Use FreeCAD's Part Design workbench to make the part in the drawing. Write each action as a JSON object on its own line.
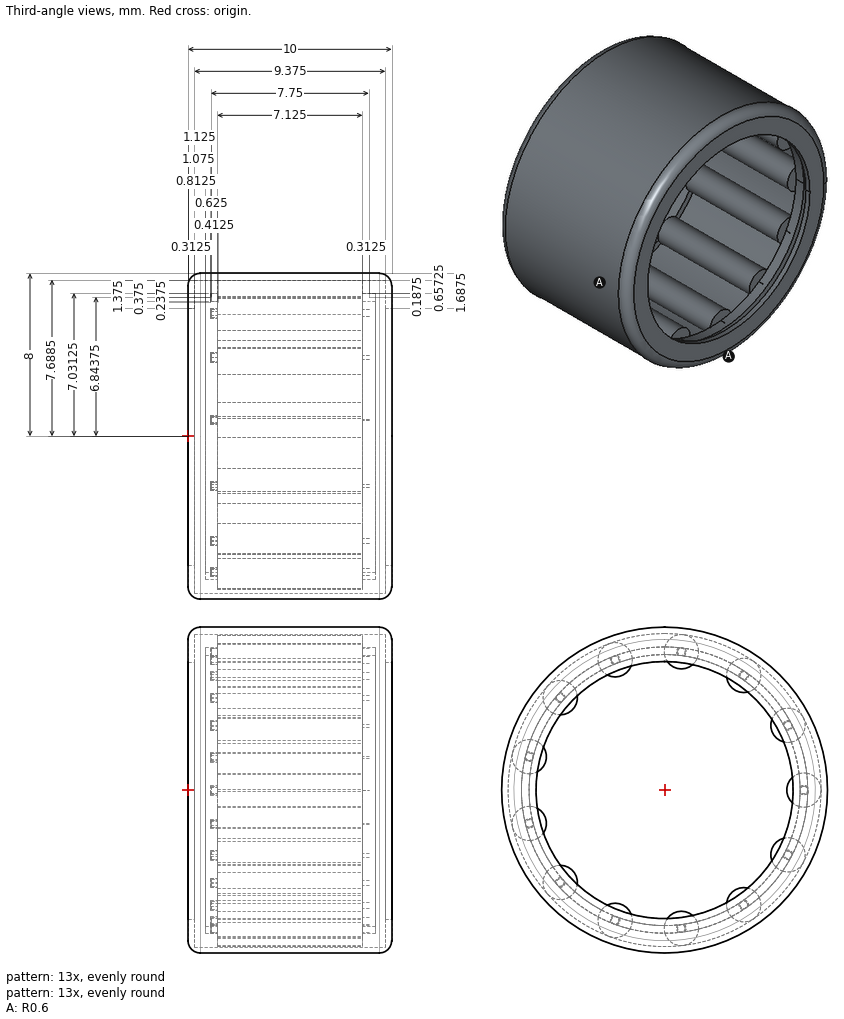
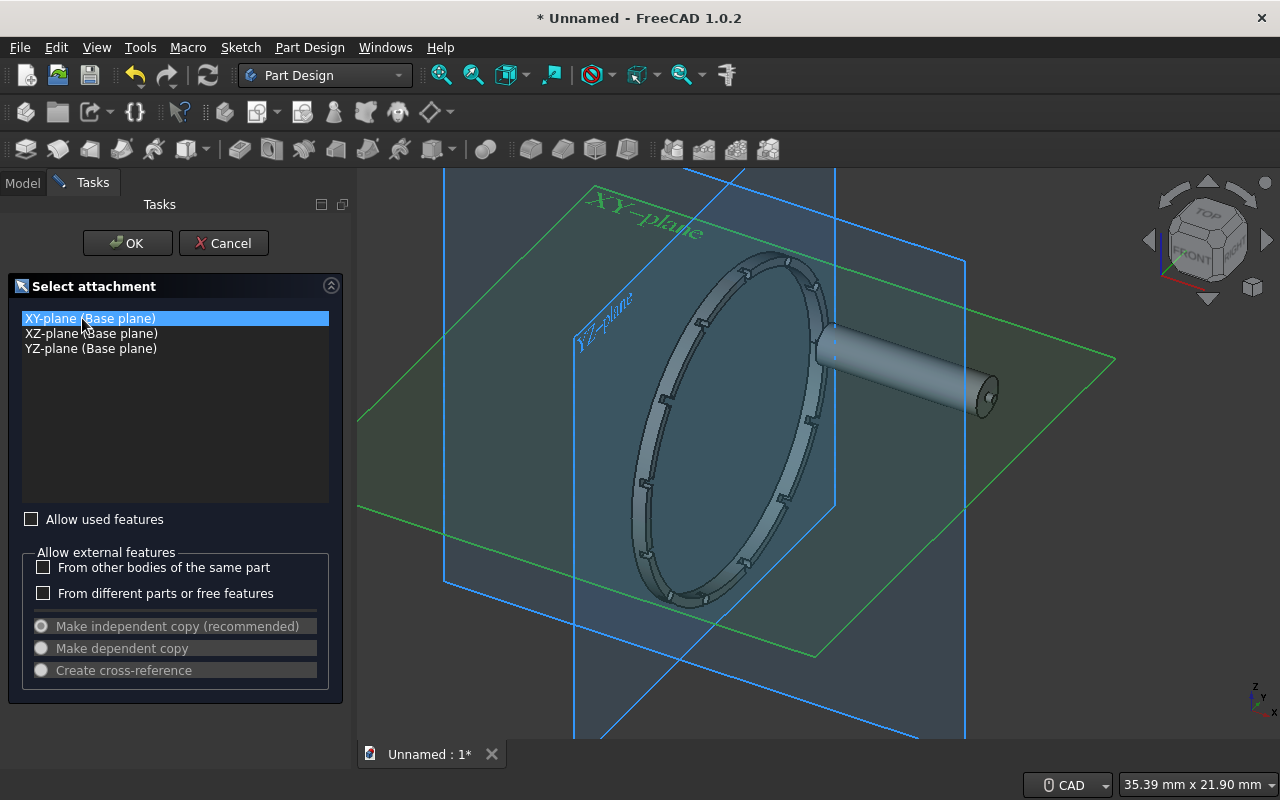
{"action": "left_click", "coordinate": [128, 243]}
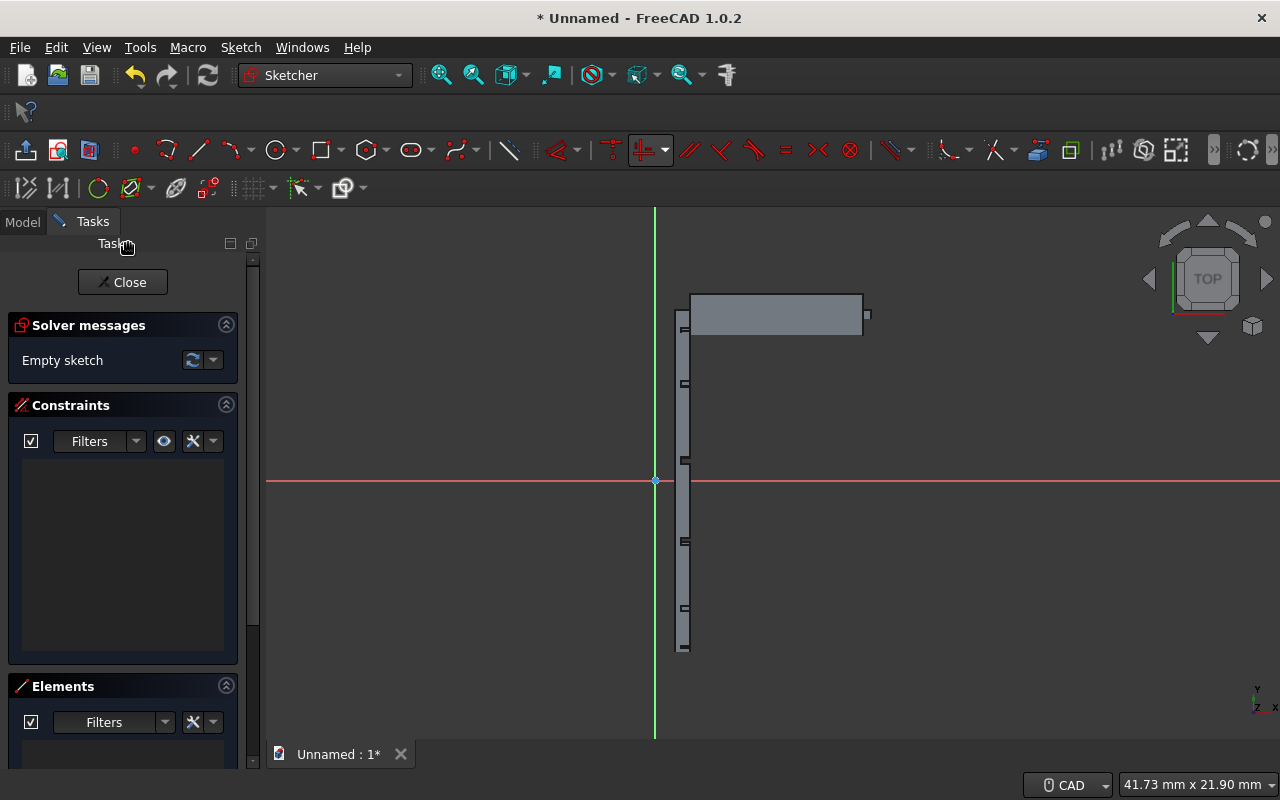
{"action": "left_click", "coordinate": [90, 150]}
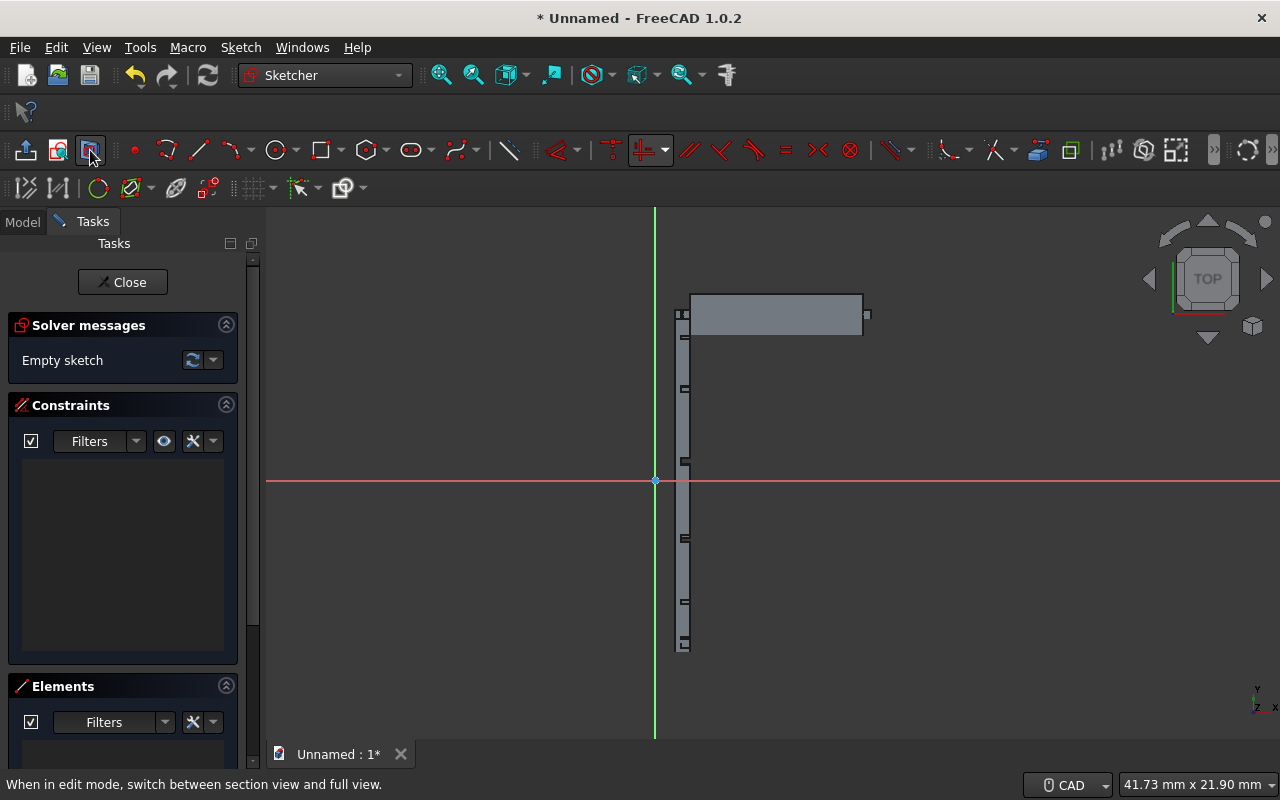
{"action": "scroll", "coordinate": [865, 275], "scroll_direction": "up", "scroll_amount": 3}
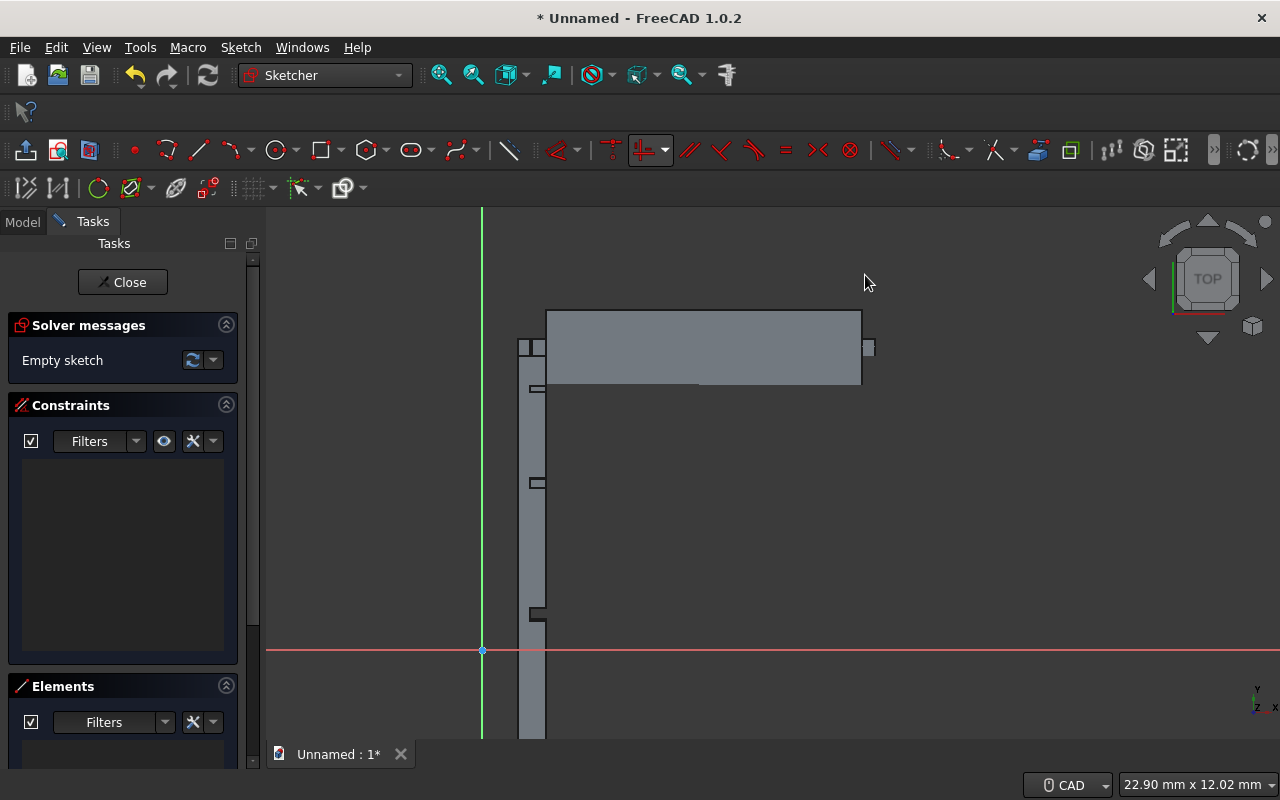
{"action": "left_click", "coordinate": [168, 150]}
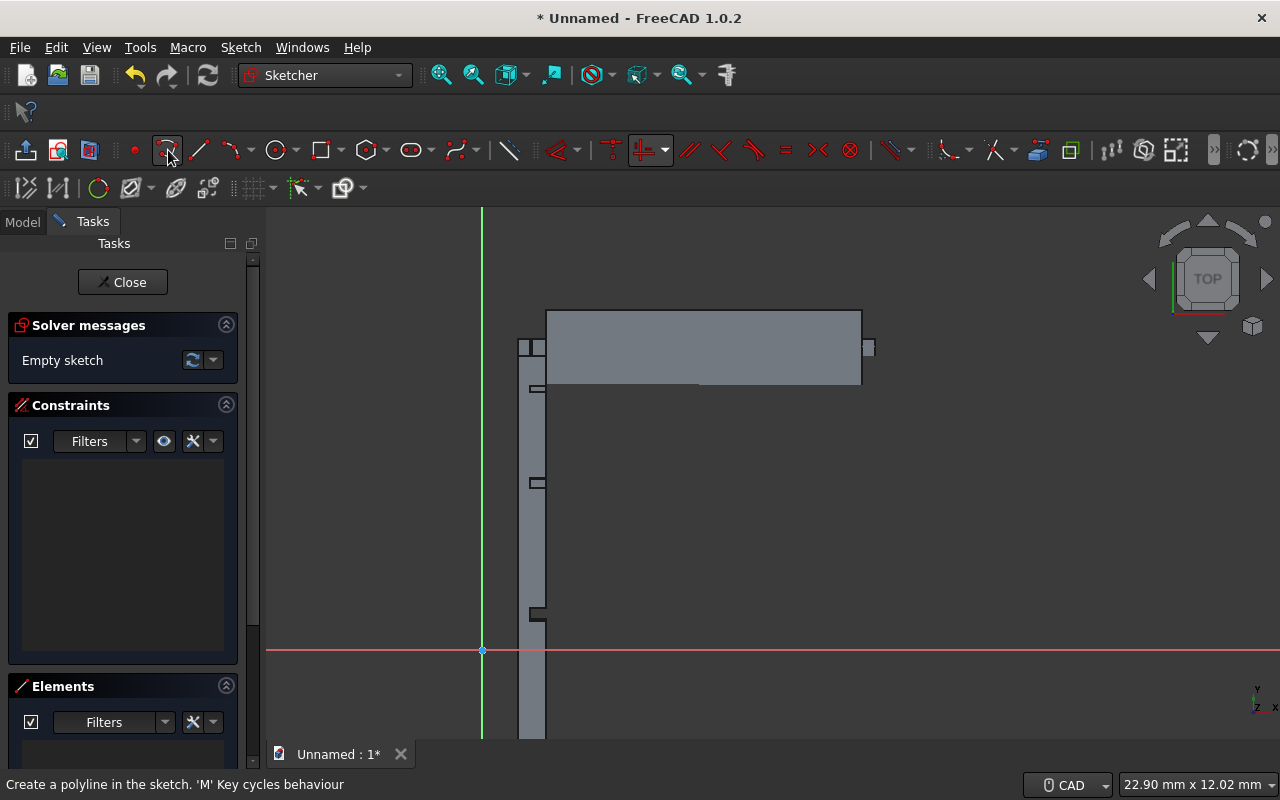
{"action": "left_click", "coordinate": [482, 371]}
{"action": "left_click", "coordinate": [496, 371]}
{"action": "left_click", "coordinate": [496, 310]}
{"action": "left_click", "coordinate": [911, 310]}
{"action": "left_click", "coordinate": [911, 371]}
{"action": "left_click", "coordinate": [925, 371]}
{"action": "left_click", "coordinate": [925, 296]}
{"action": "left_click", "coordinate": [491, 296]}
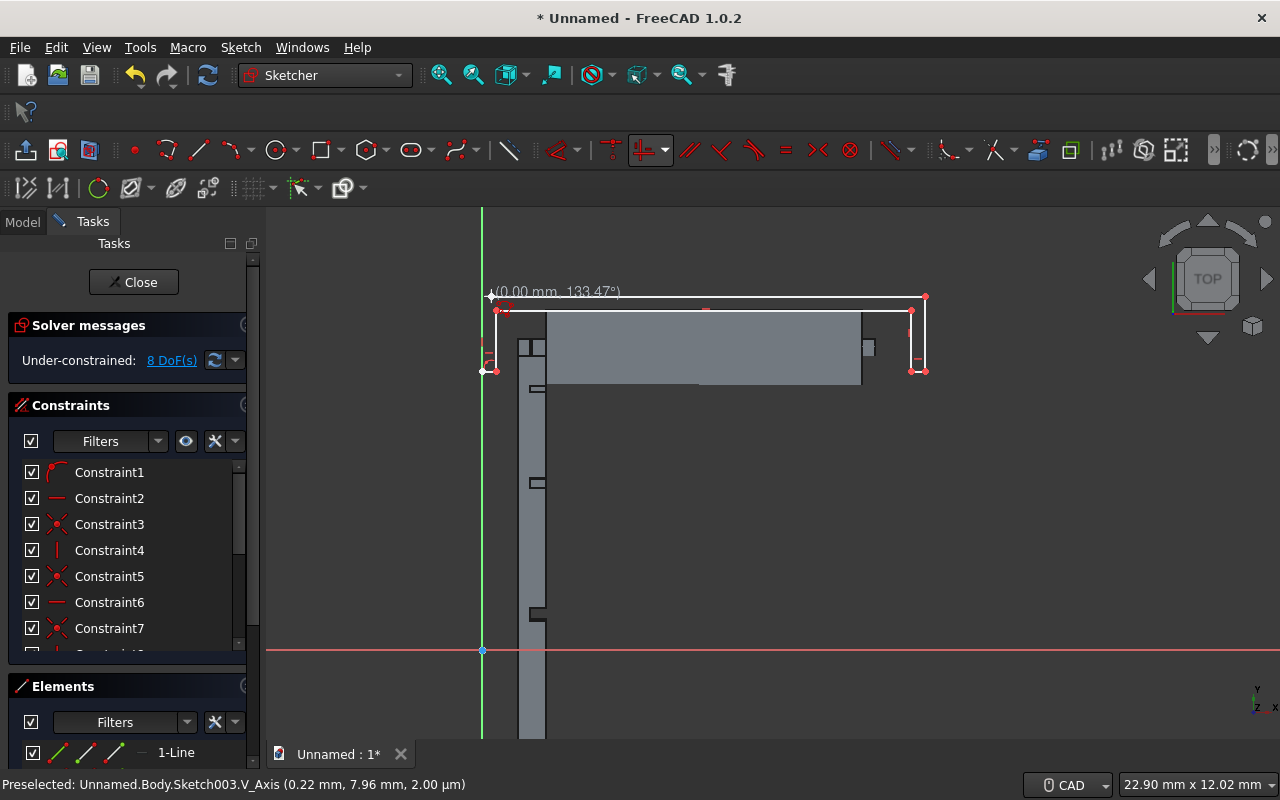
{"action": "scroll", "coordinate": [482, 371], "scroll_direction": "up", "scroll_amount": 5}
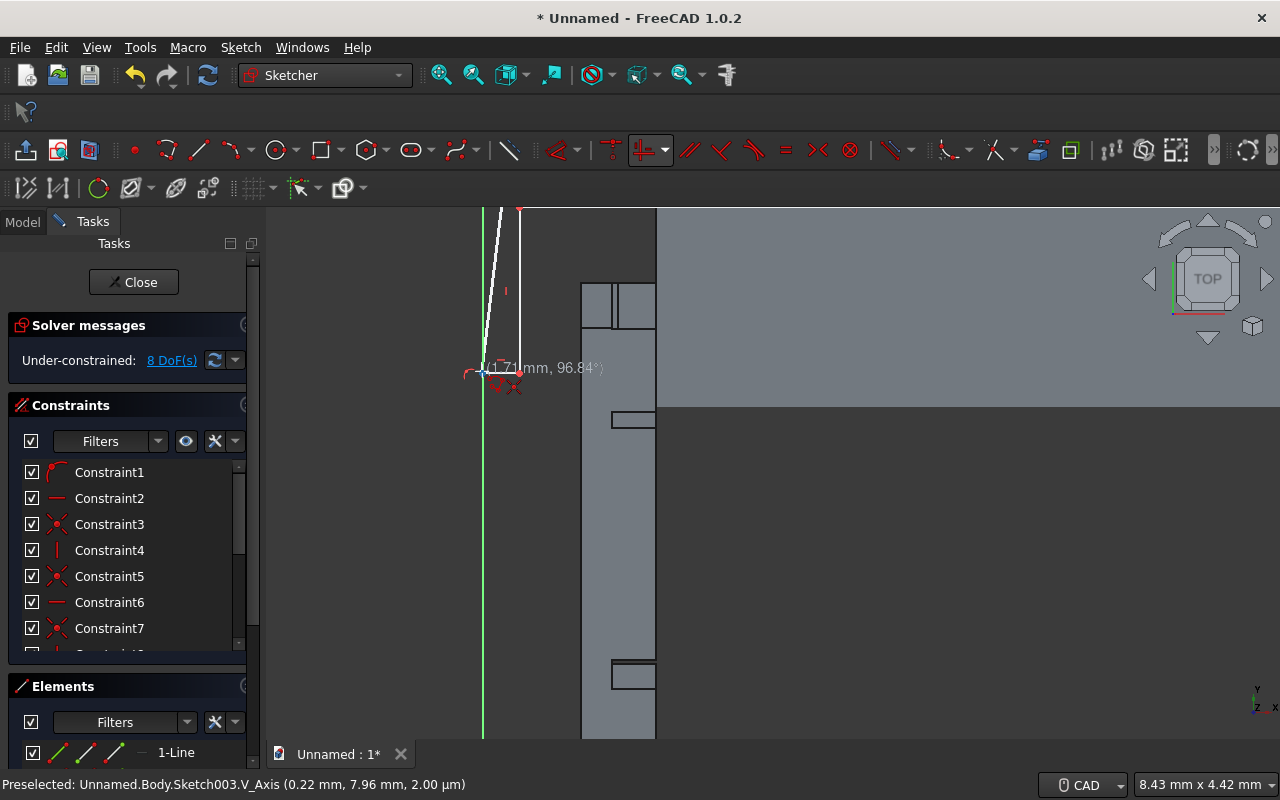
{"action": "left_click", "coordinate": [483, 373]}
{"action": "key", "text": "Escape"}
{"action": "key", "text": "Escape"}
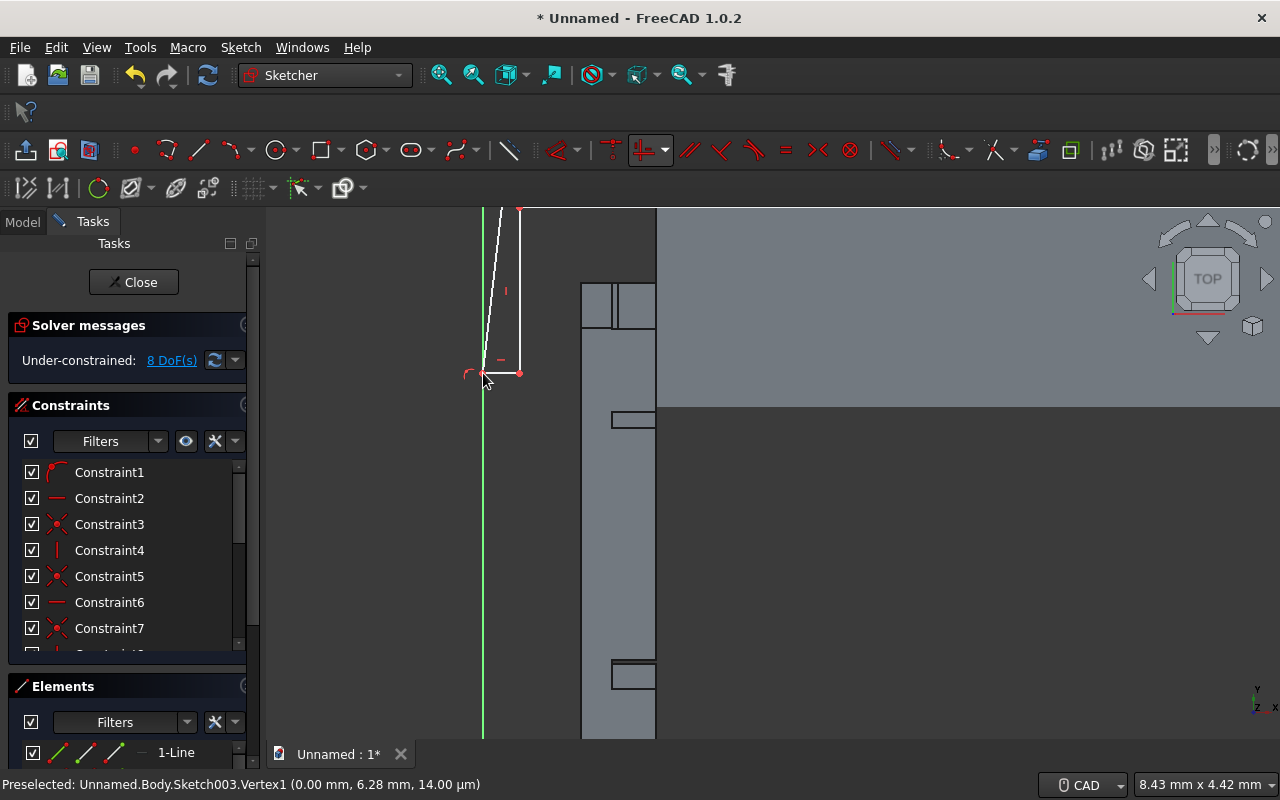
{"action": "left_click", "coordinate": [497, 251]}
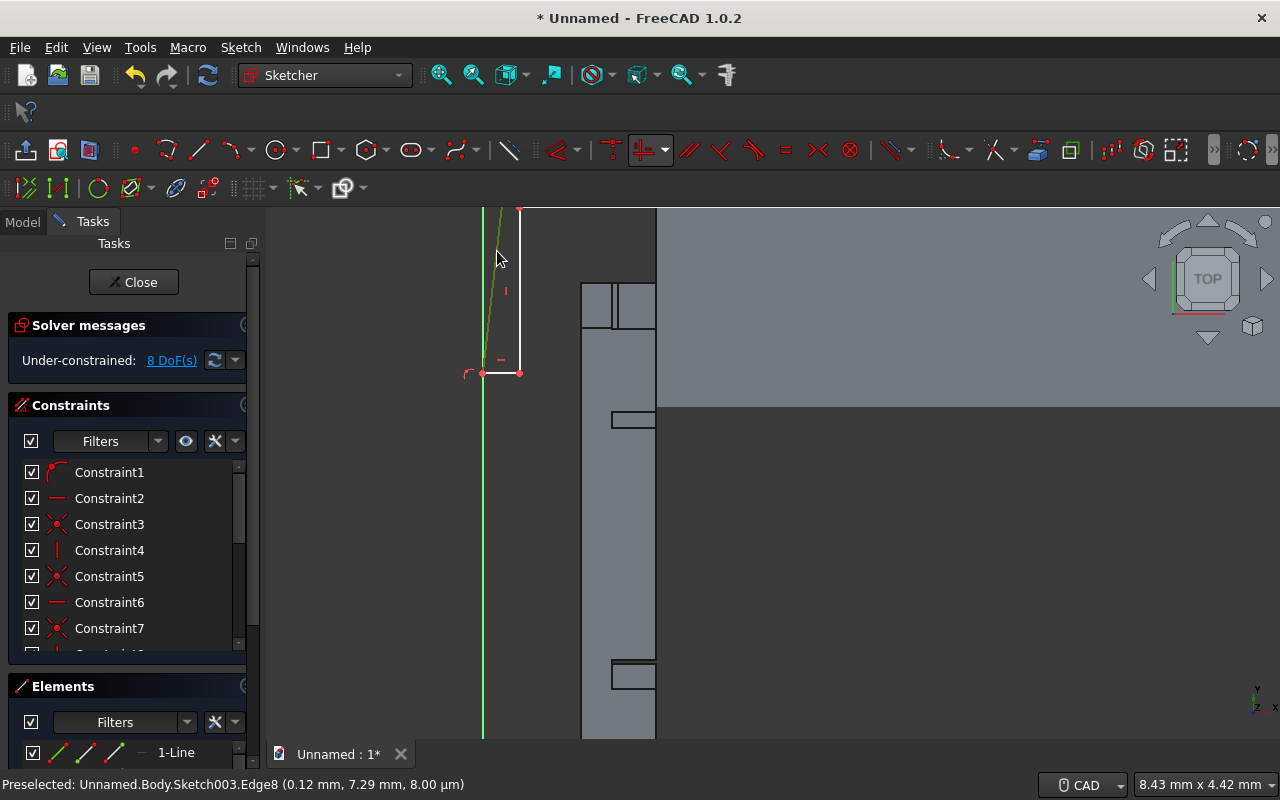
{"action": "left_click", "coordinate": [668, 150]}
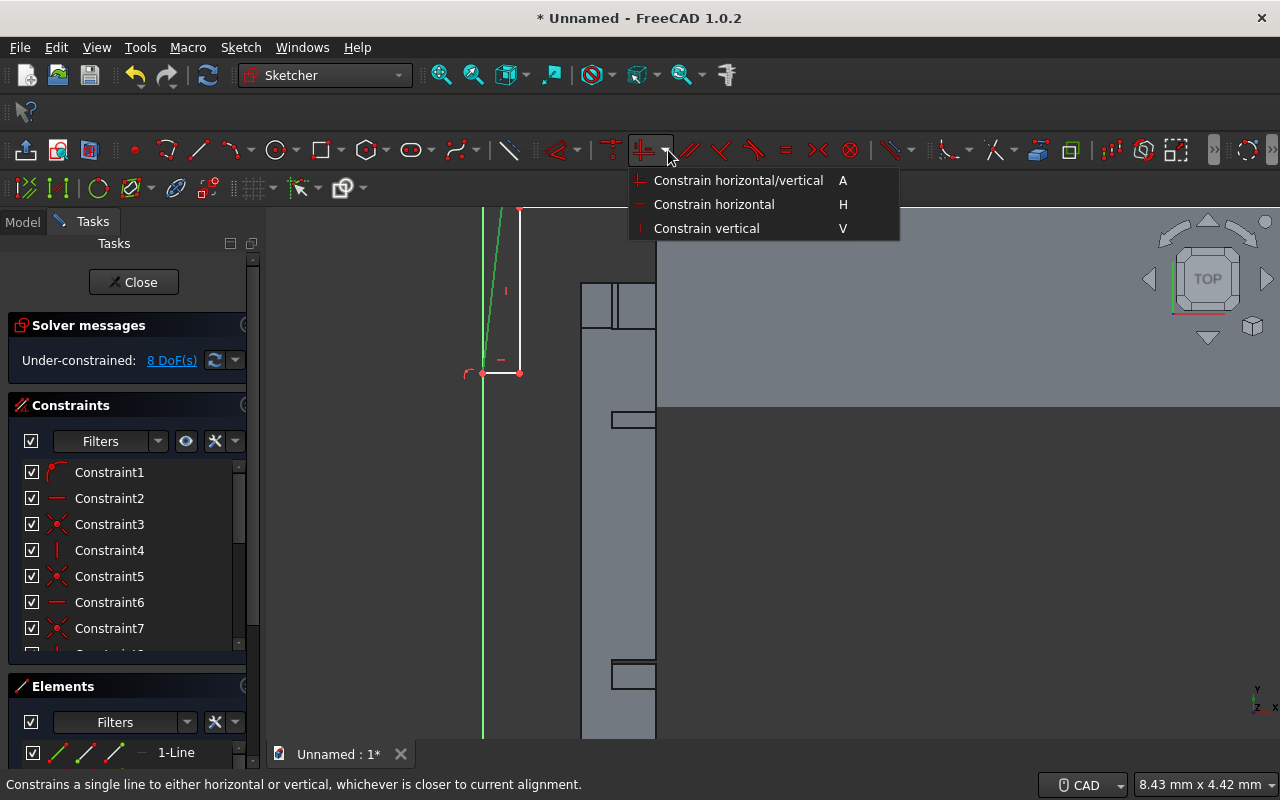
{"action": "left_click", "coordinate": [764, 228]}